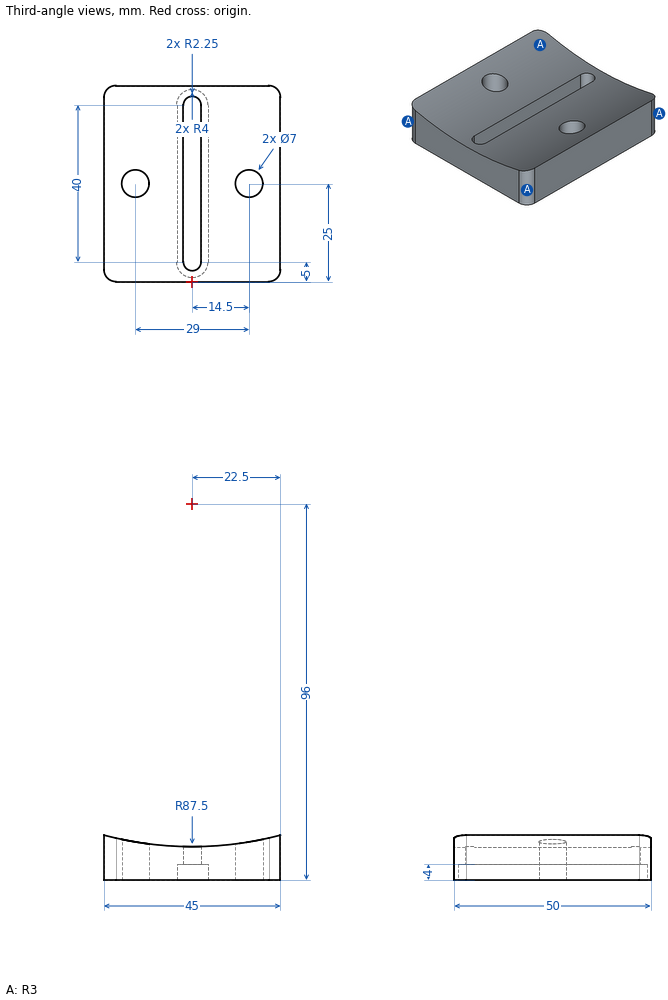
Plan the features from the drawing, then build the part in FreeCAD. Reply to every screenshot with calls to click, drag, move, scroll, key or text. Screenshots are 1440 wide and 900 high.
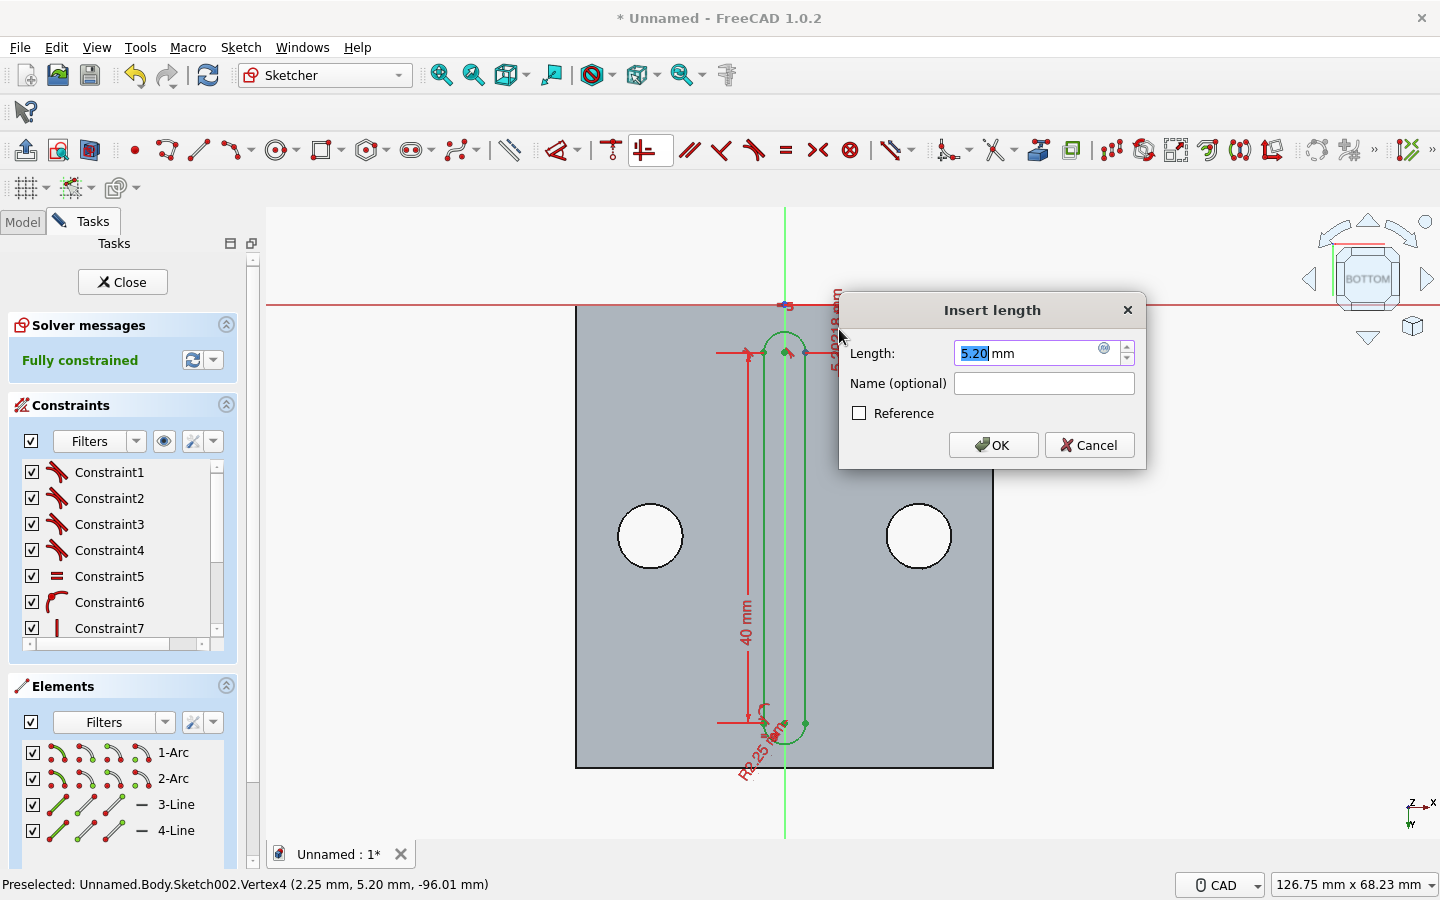
text(5)
key(Return)
key(Escape)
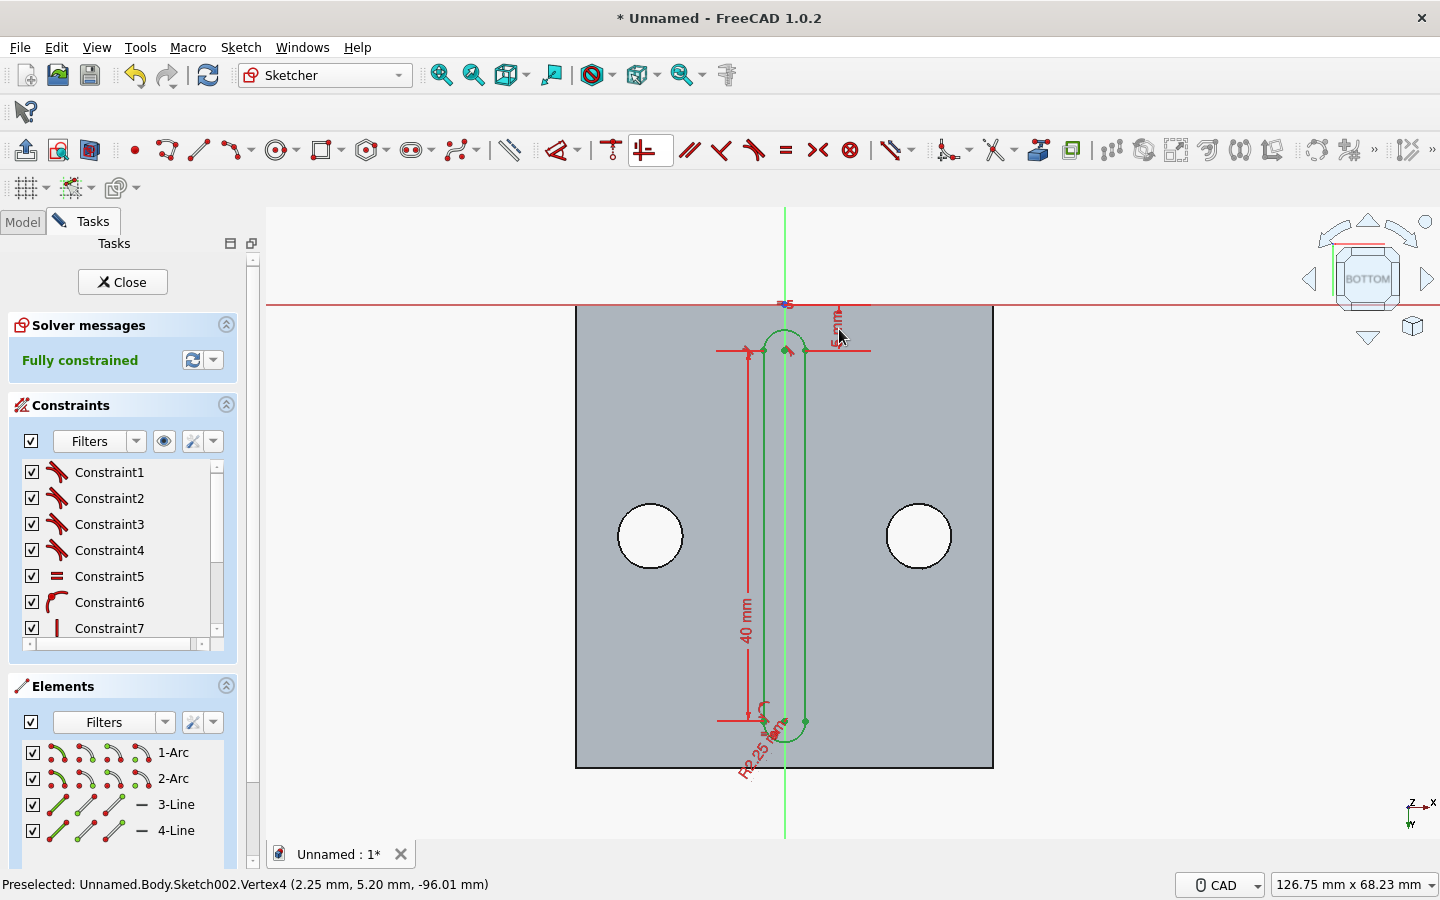
click(123, 282)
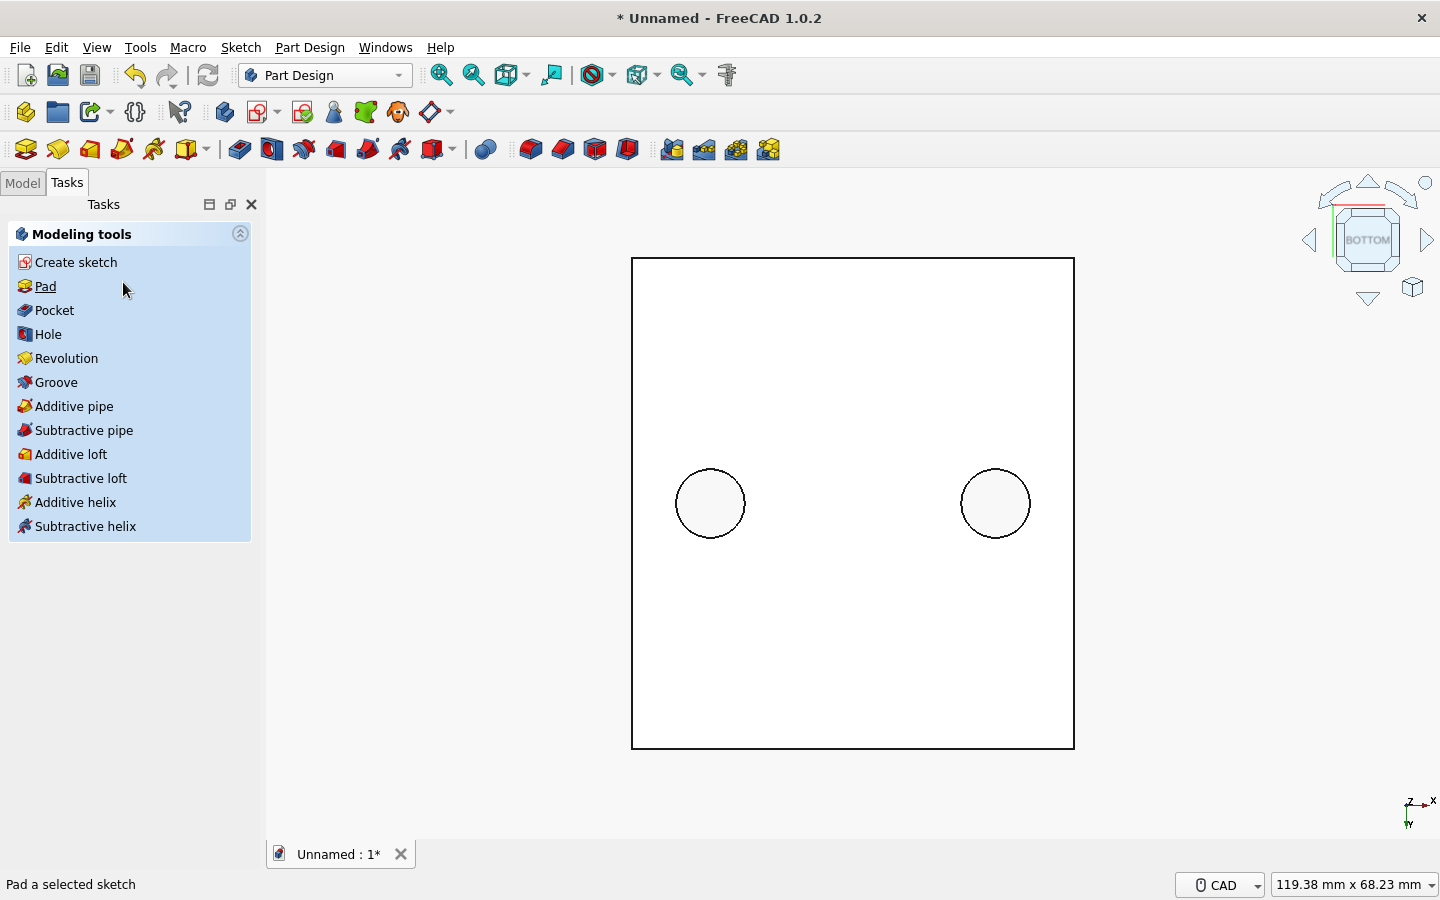
click(240, 150)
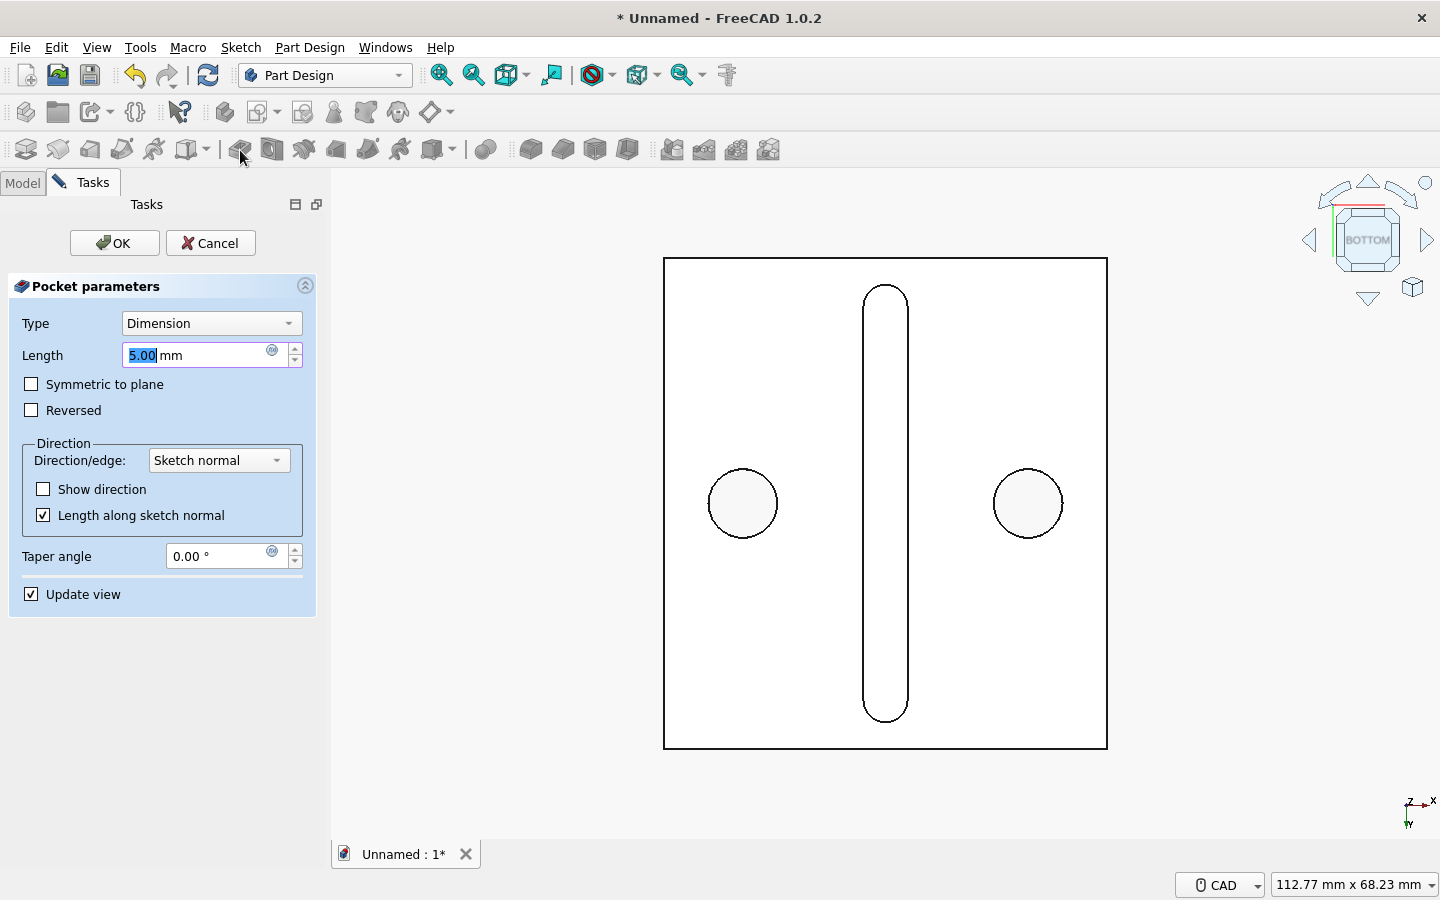
click(212, 324)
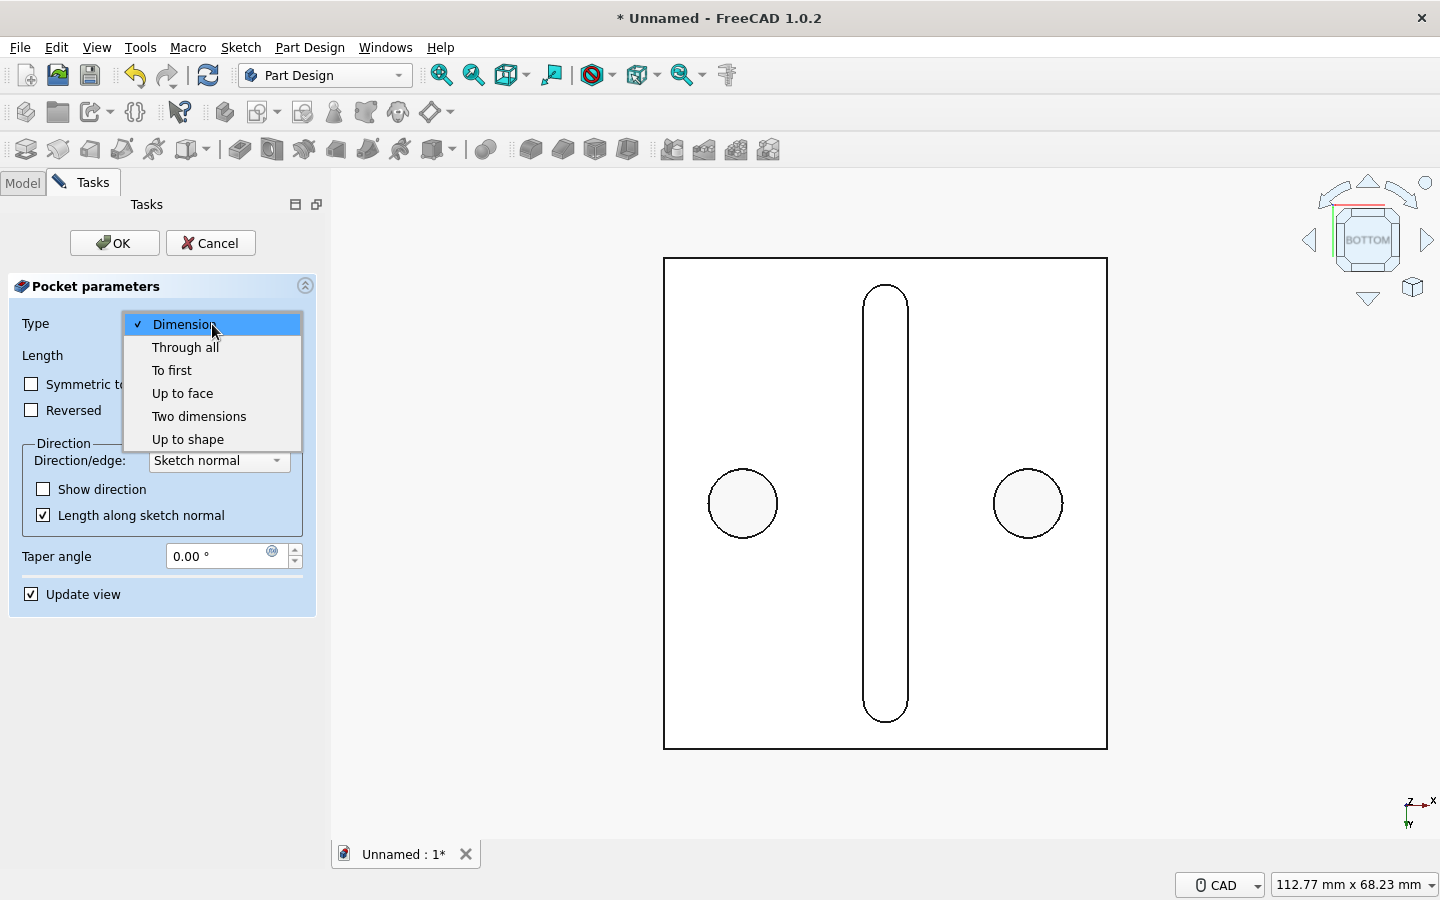
click(212, 348)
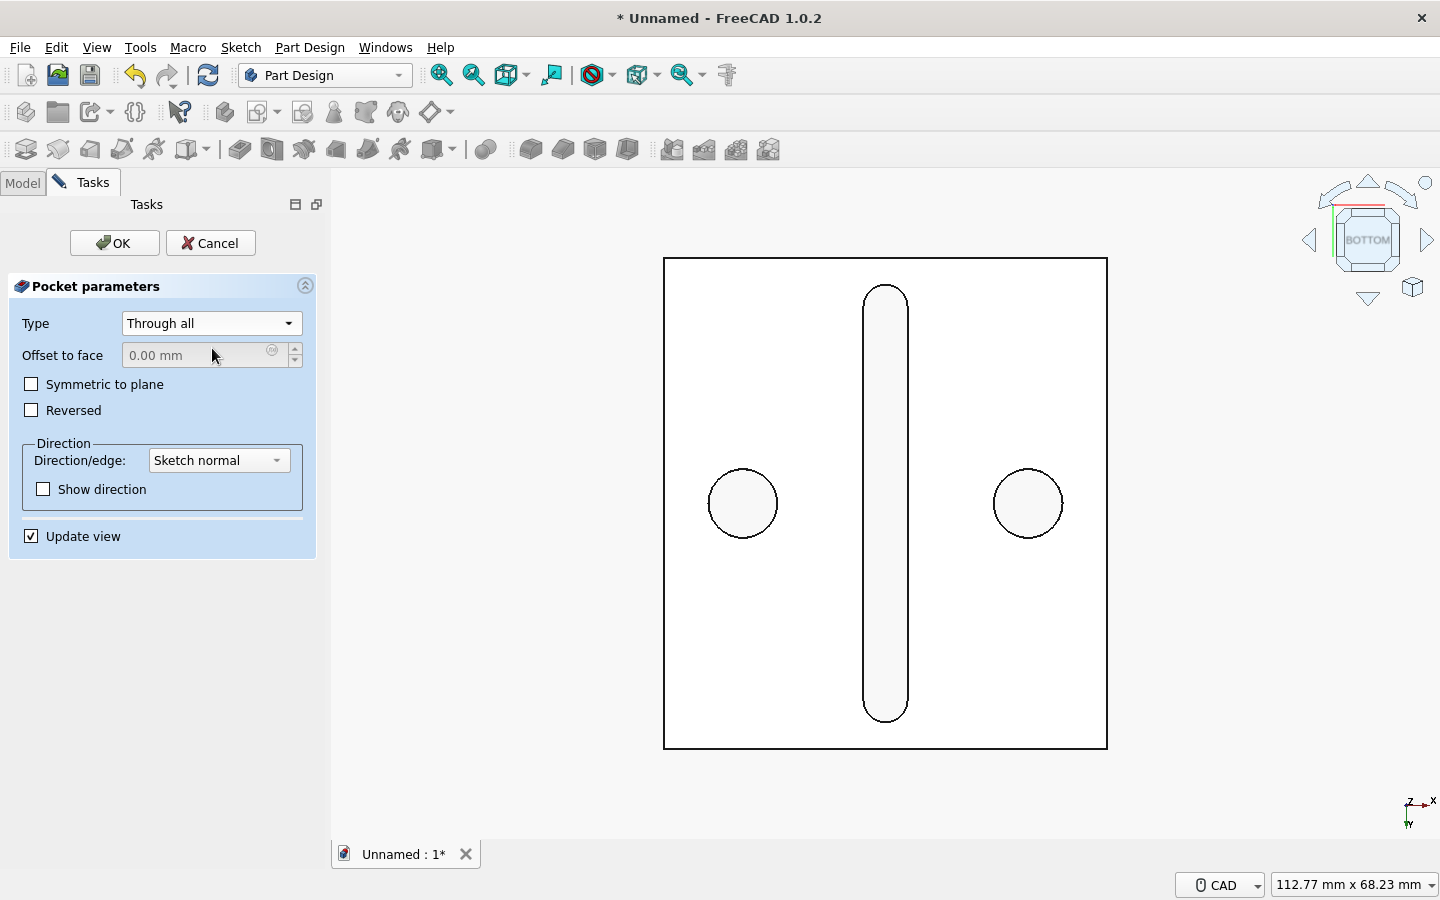
click(115, 243)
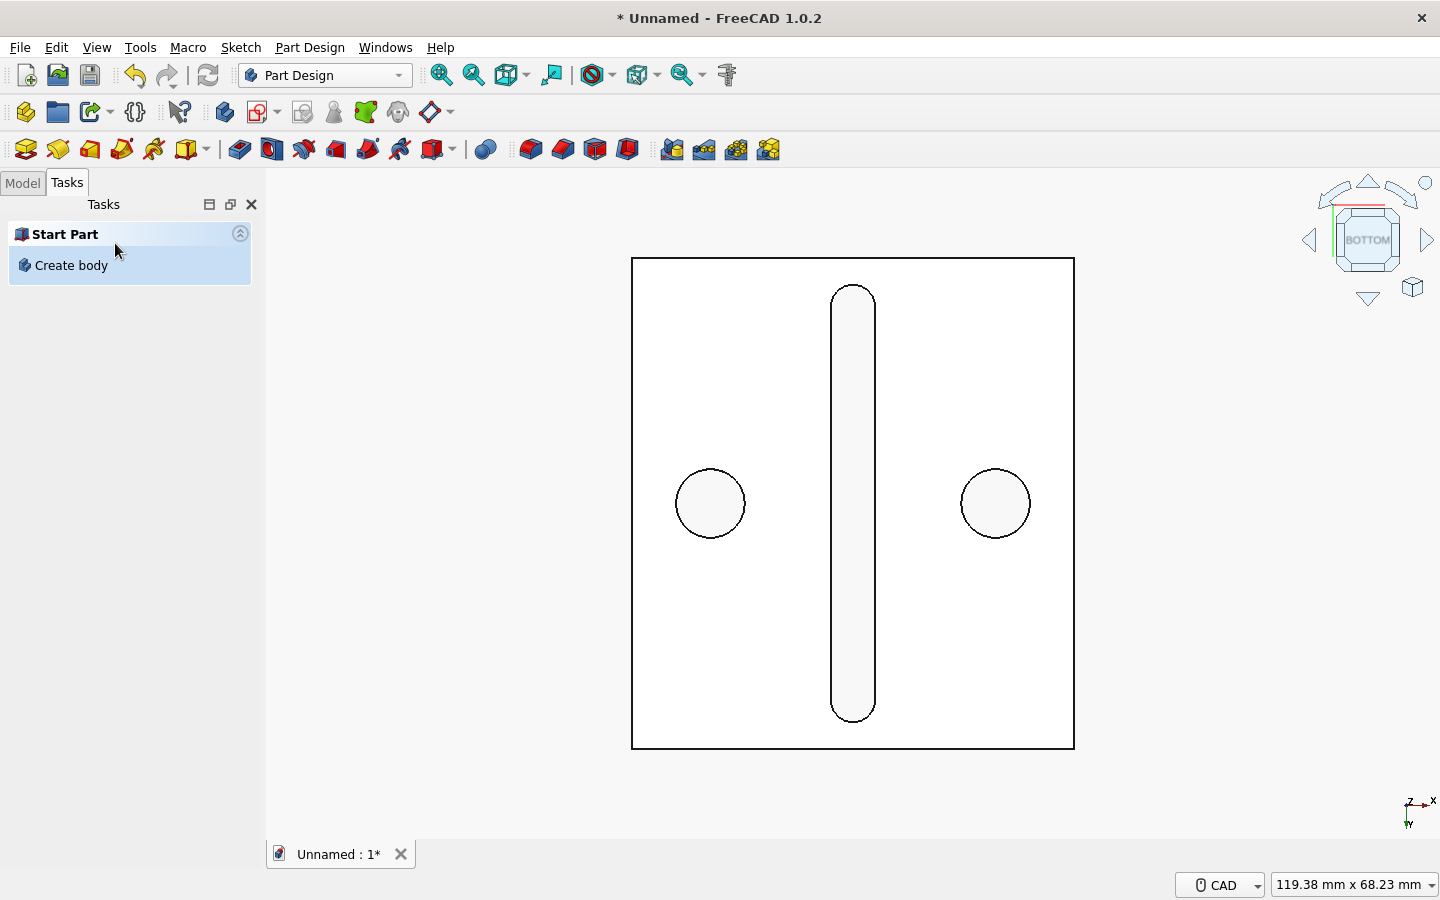
click(727, 643)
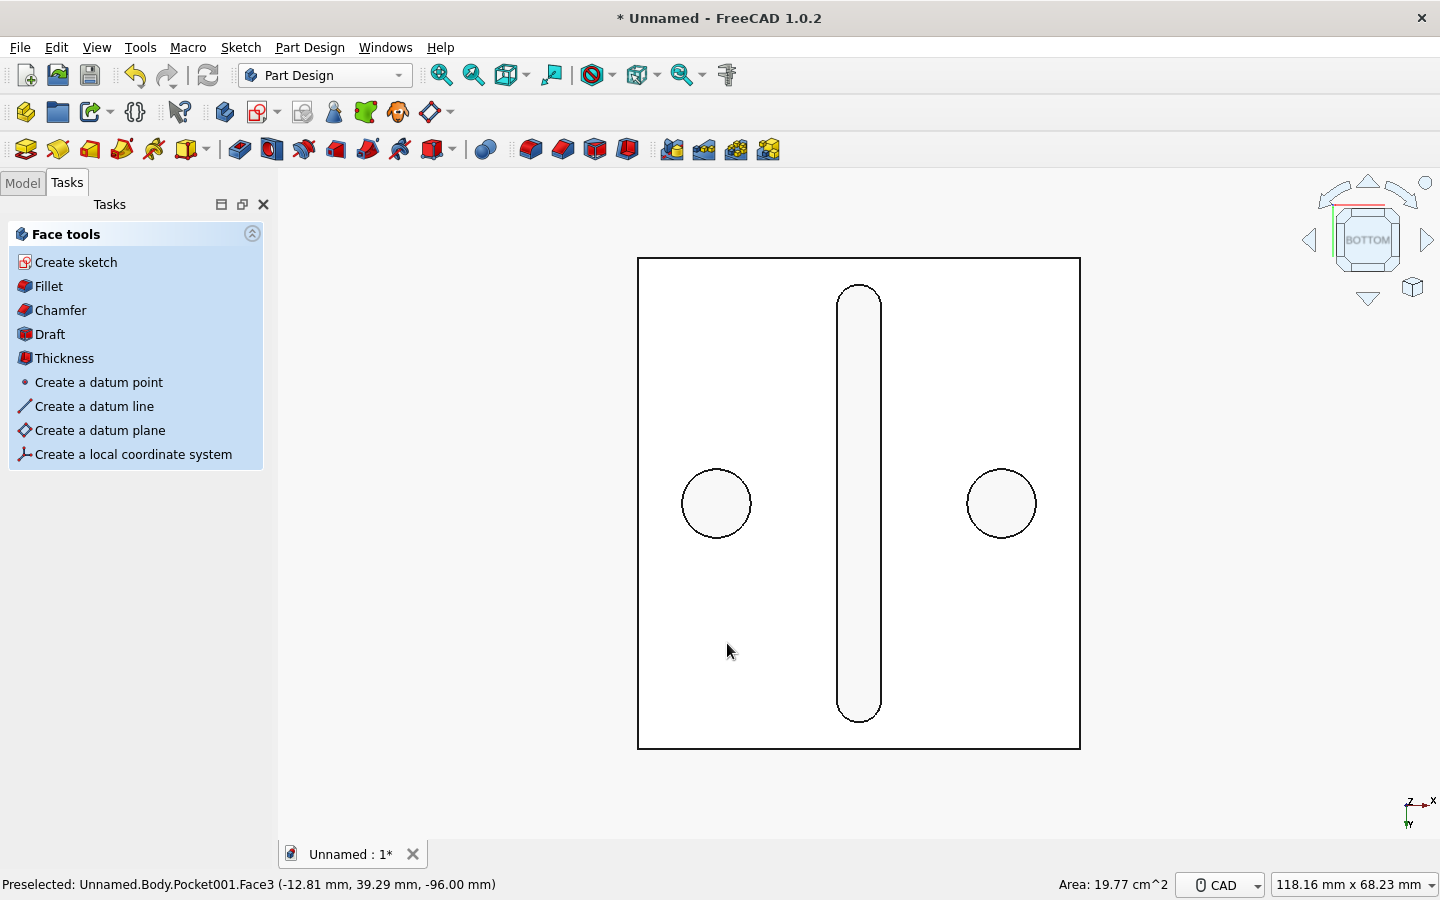
click(258, 112)